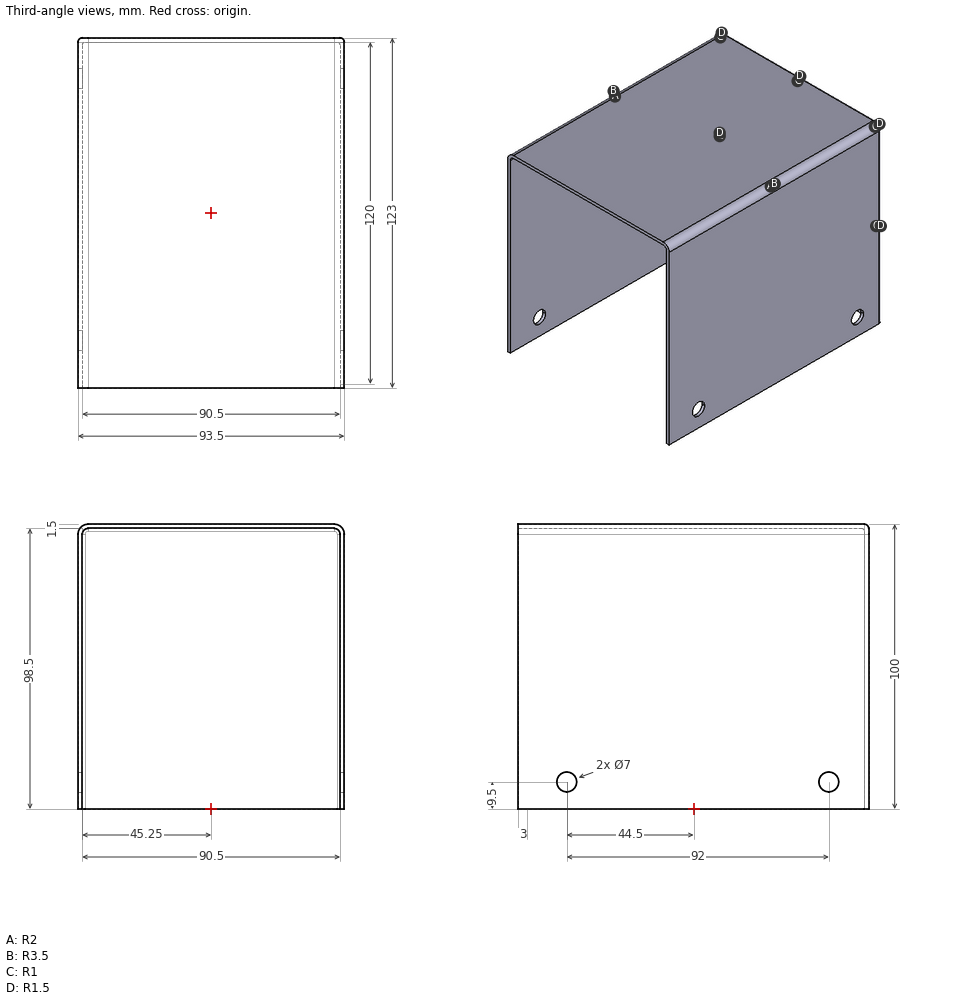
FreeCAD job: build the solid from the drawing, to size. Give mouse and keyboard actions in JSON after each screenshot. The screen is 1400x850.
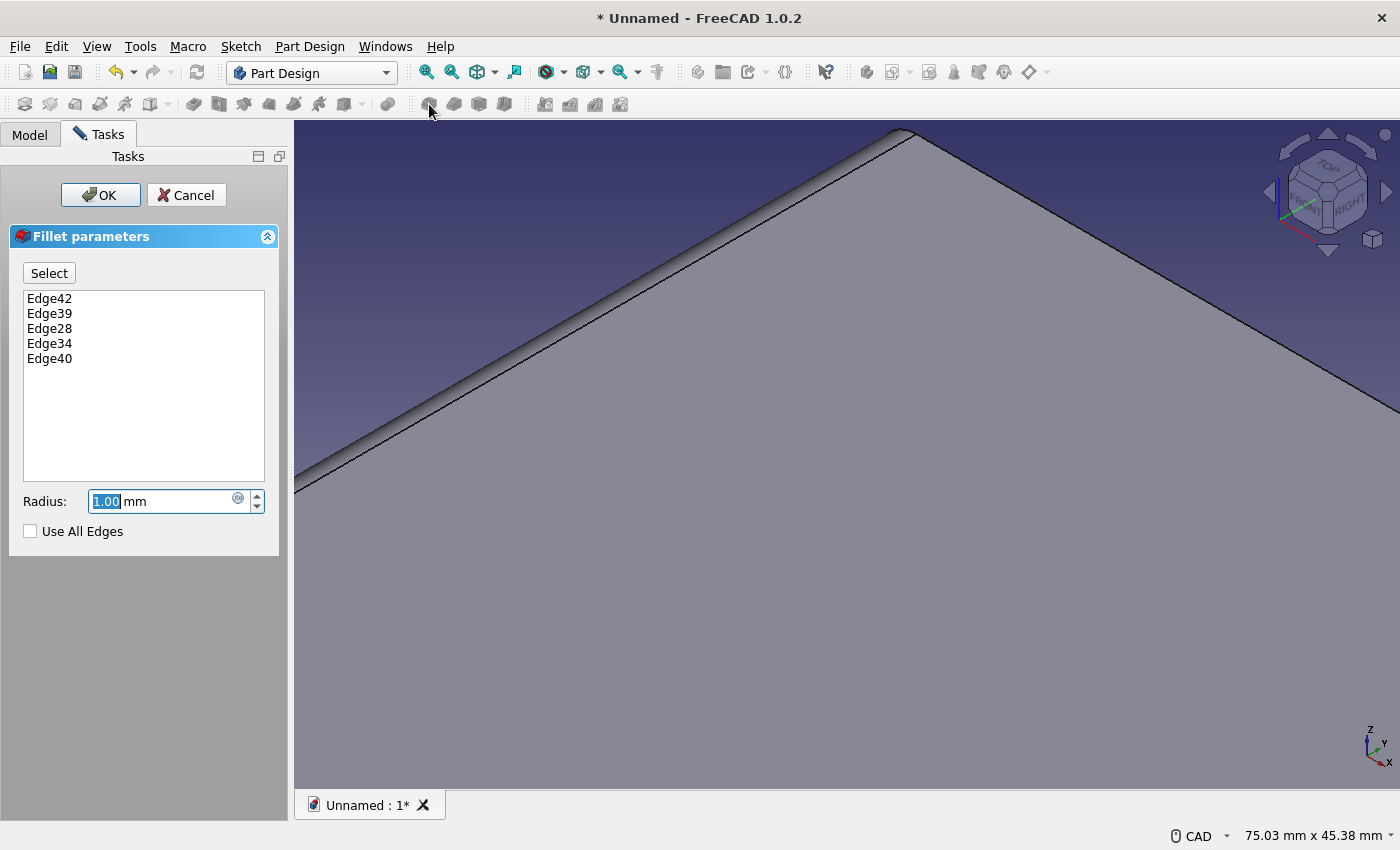
{"action": "type", "text": "1"}
{"action": "key", "text": "Tab"}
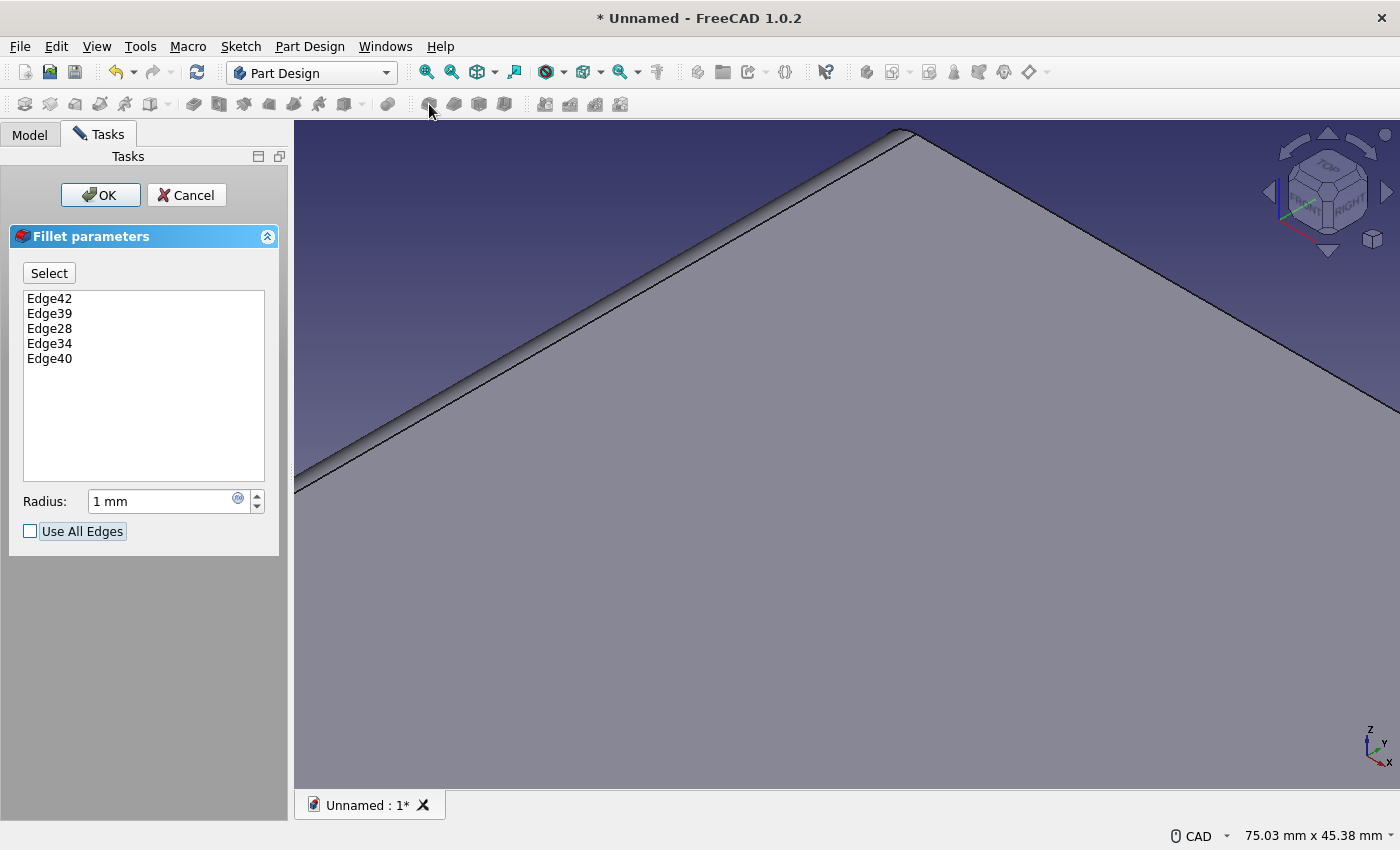
{"action": "left_click", "coordinate": [101, 195]}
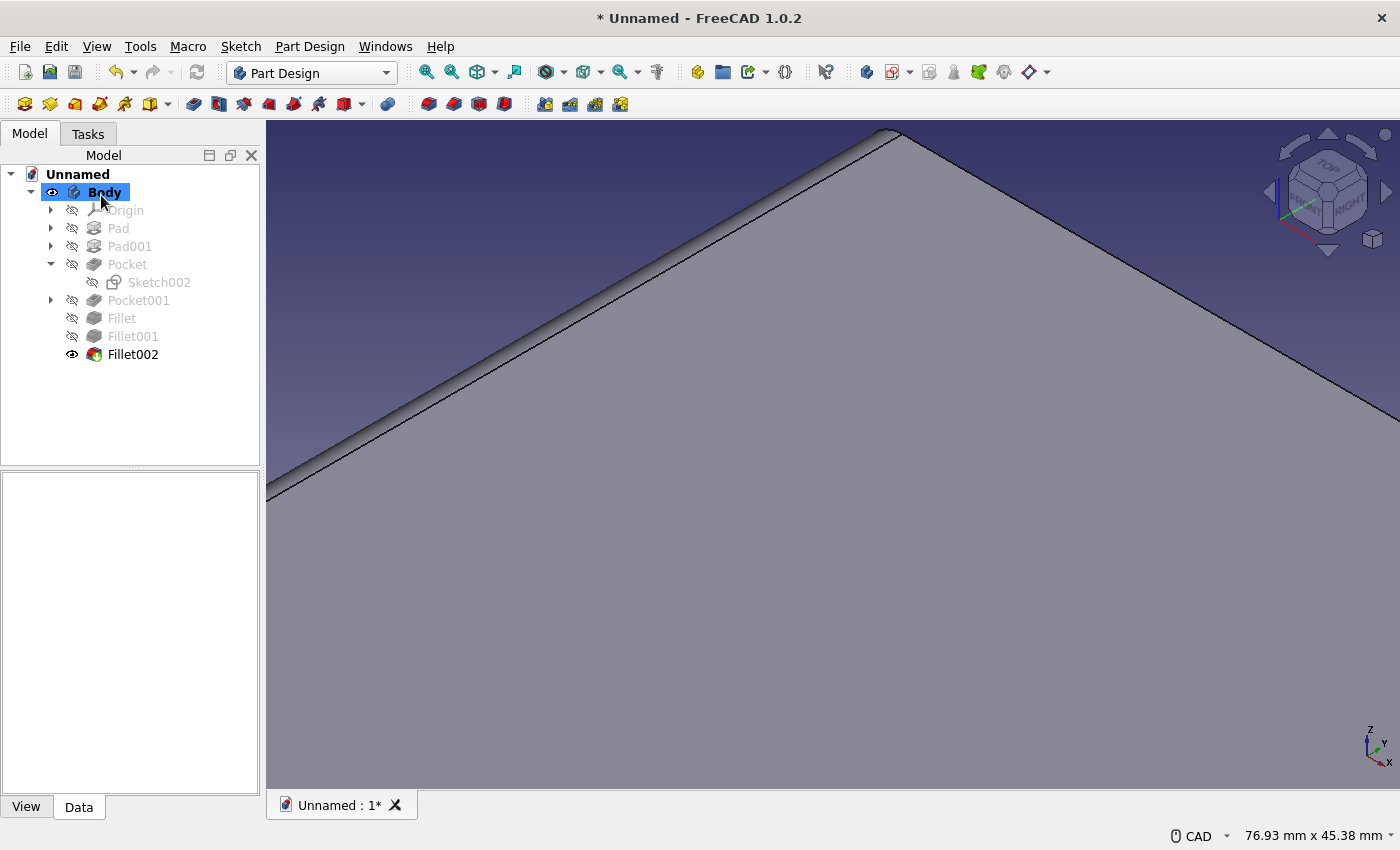
{"action": "left_click", "coordinate": [427, 72]}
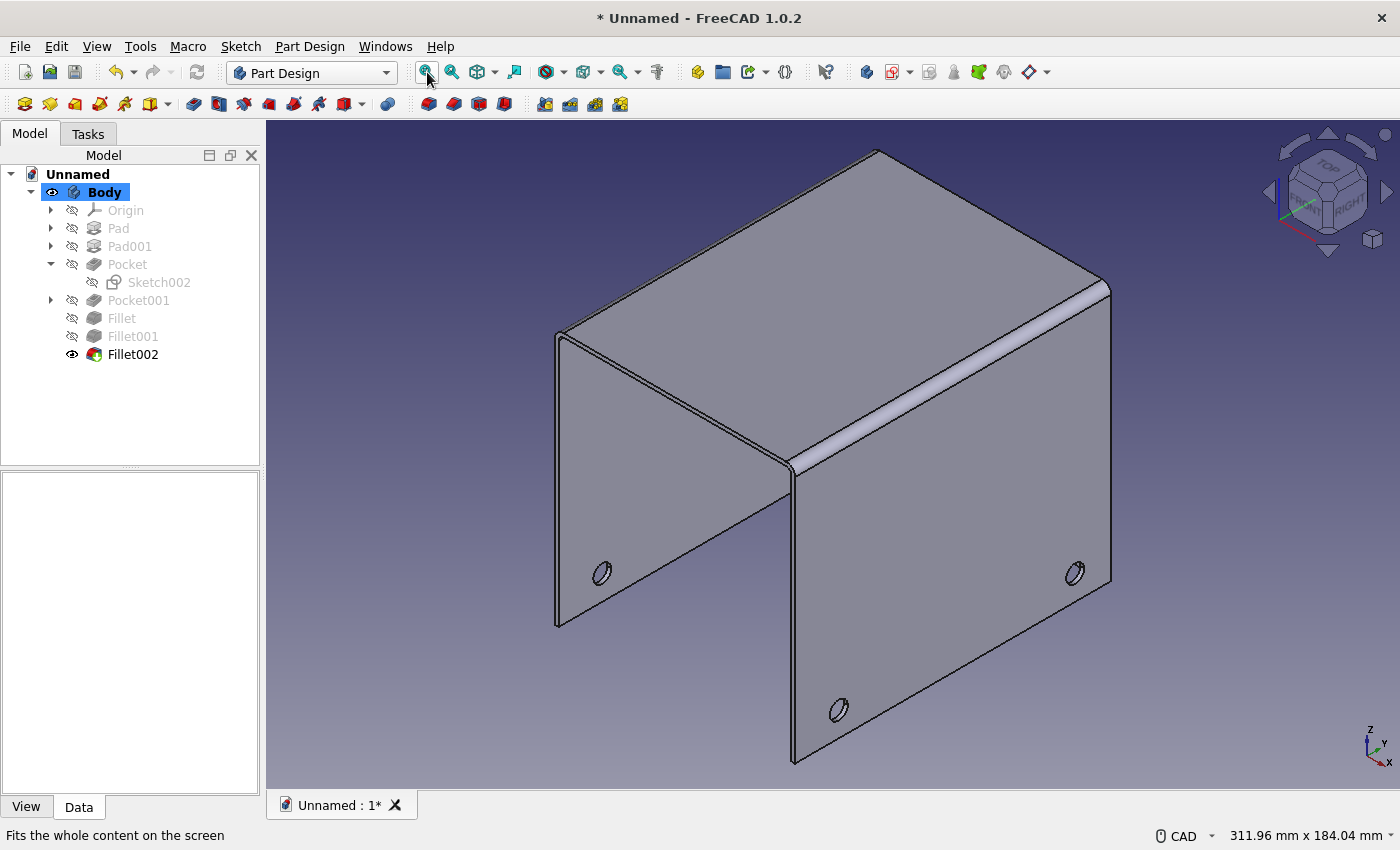
{"action": "left_click", "coordinate": [1111, 290]}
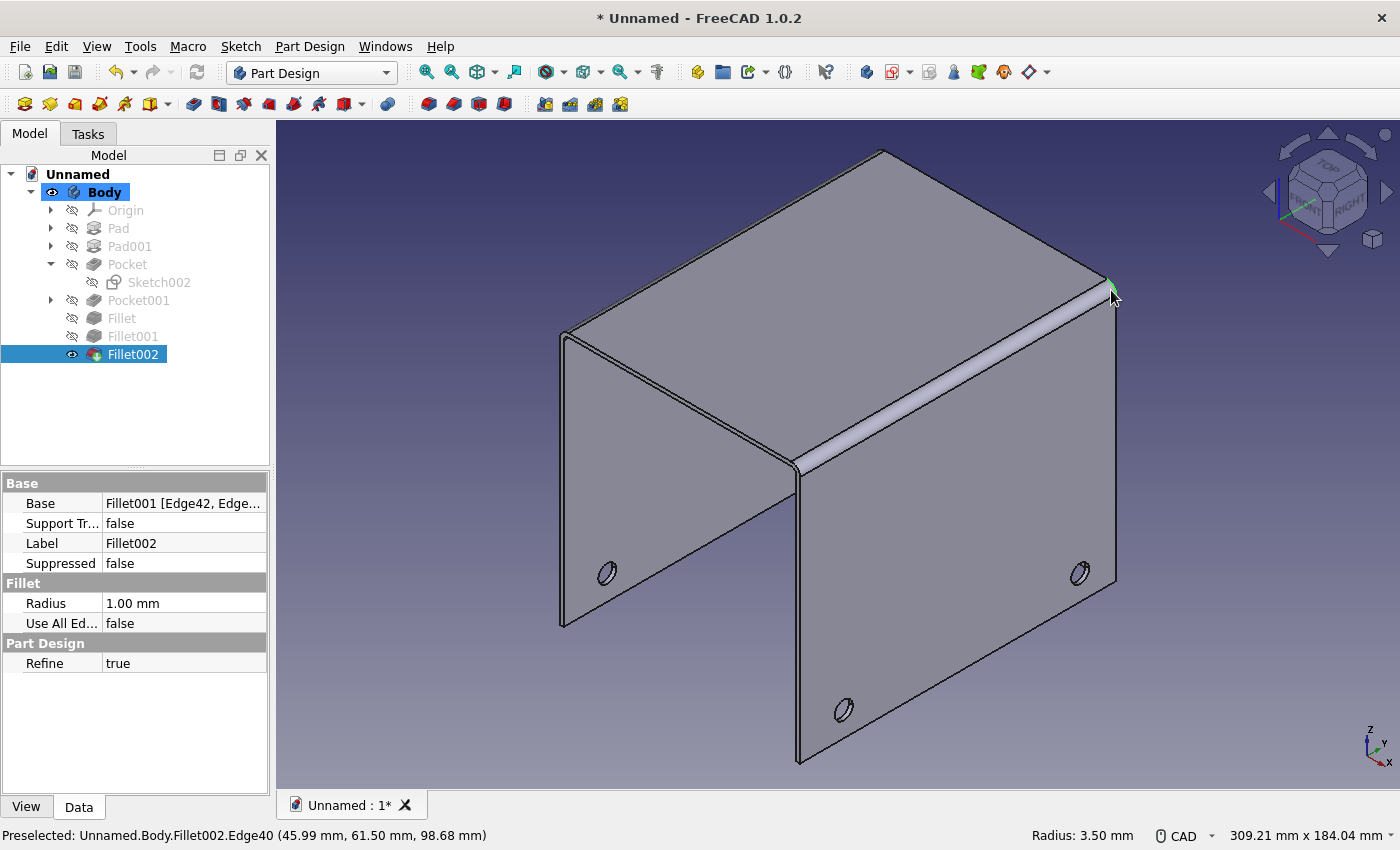
{"action": "key", "text": "2"}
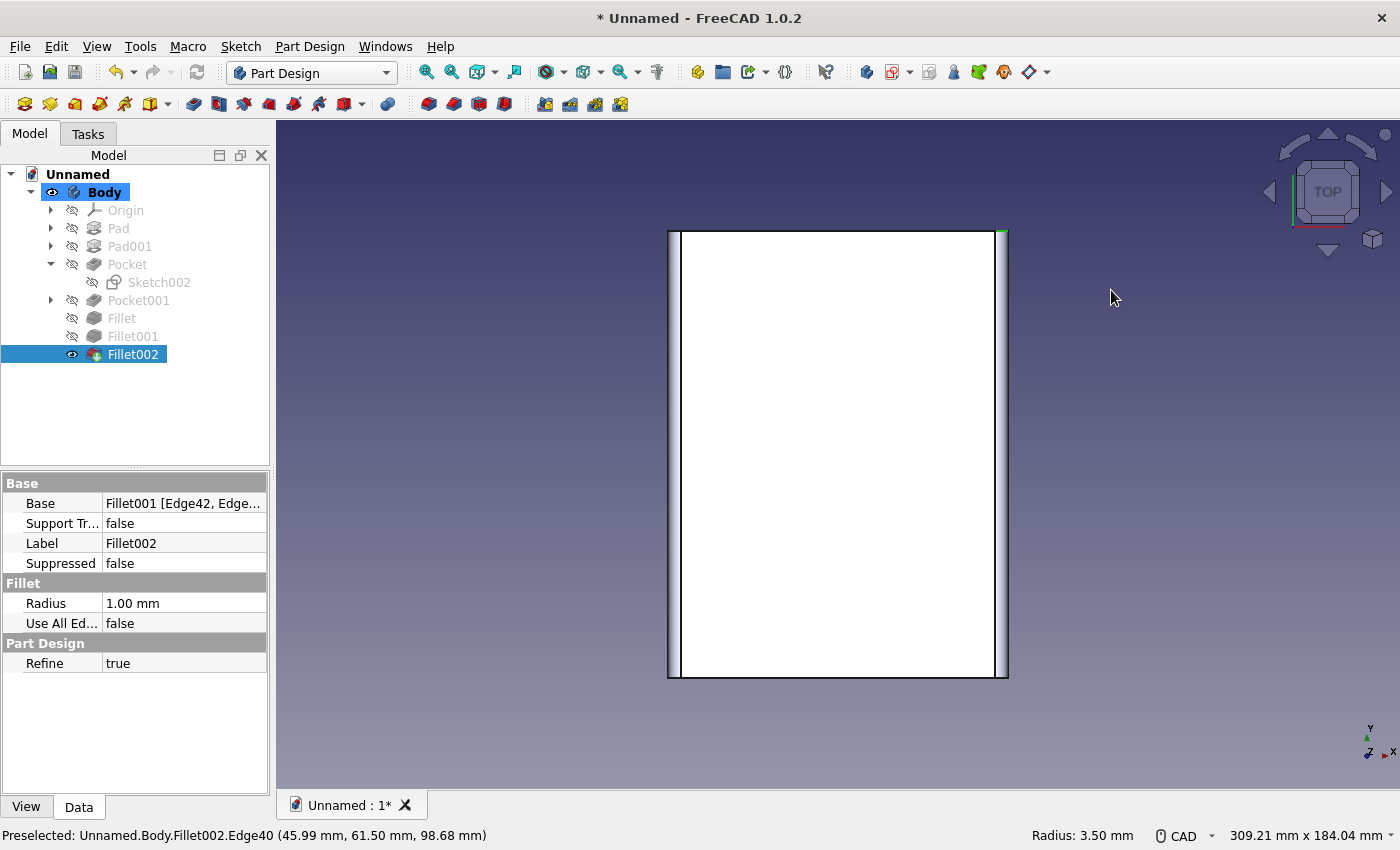
{"action": "left_click", "coordinate": [672, 230], "text": "ctrl"}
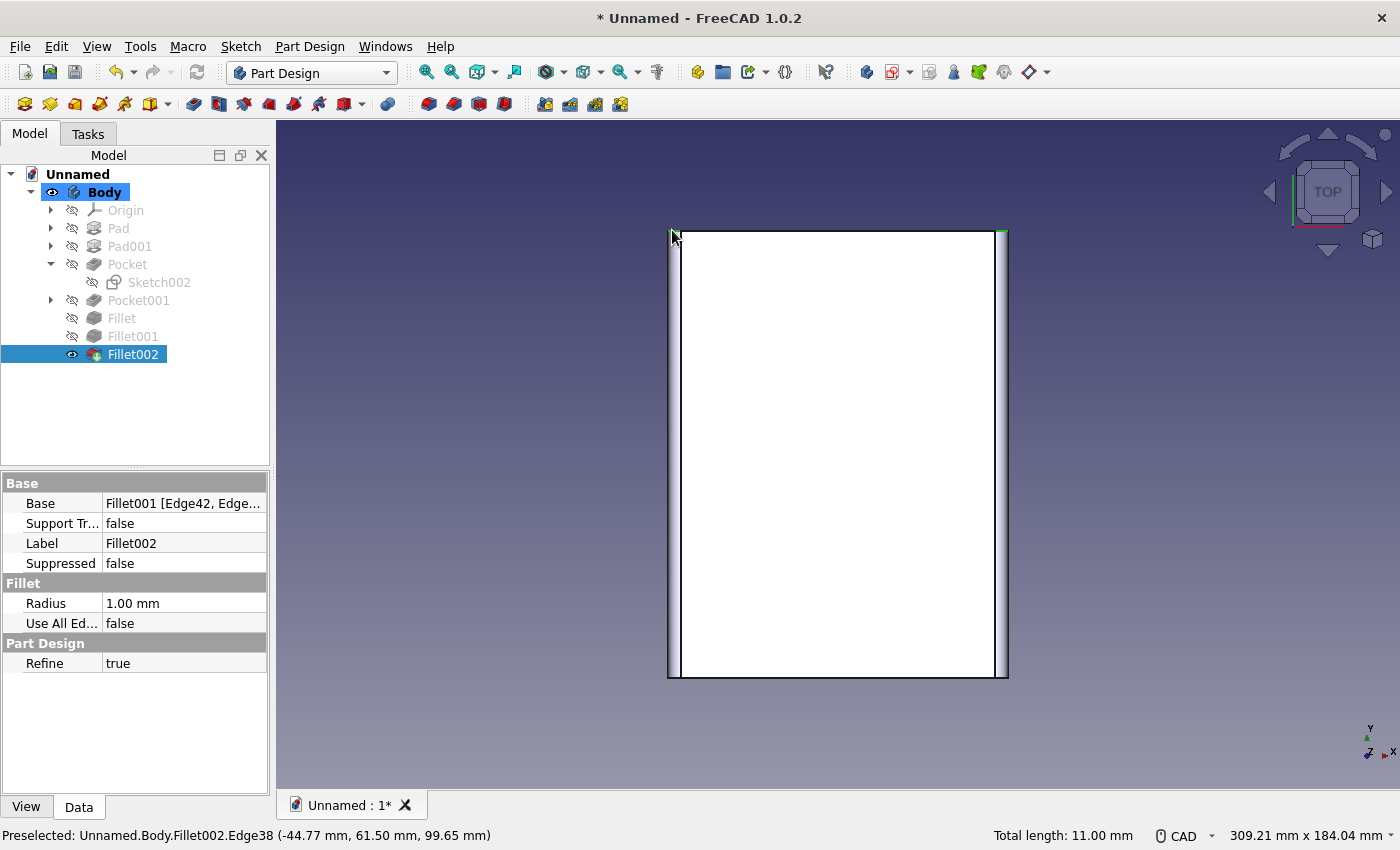
{"action": "left_click", "coordinate": [838, 230], "text": "ctrl"}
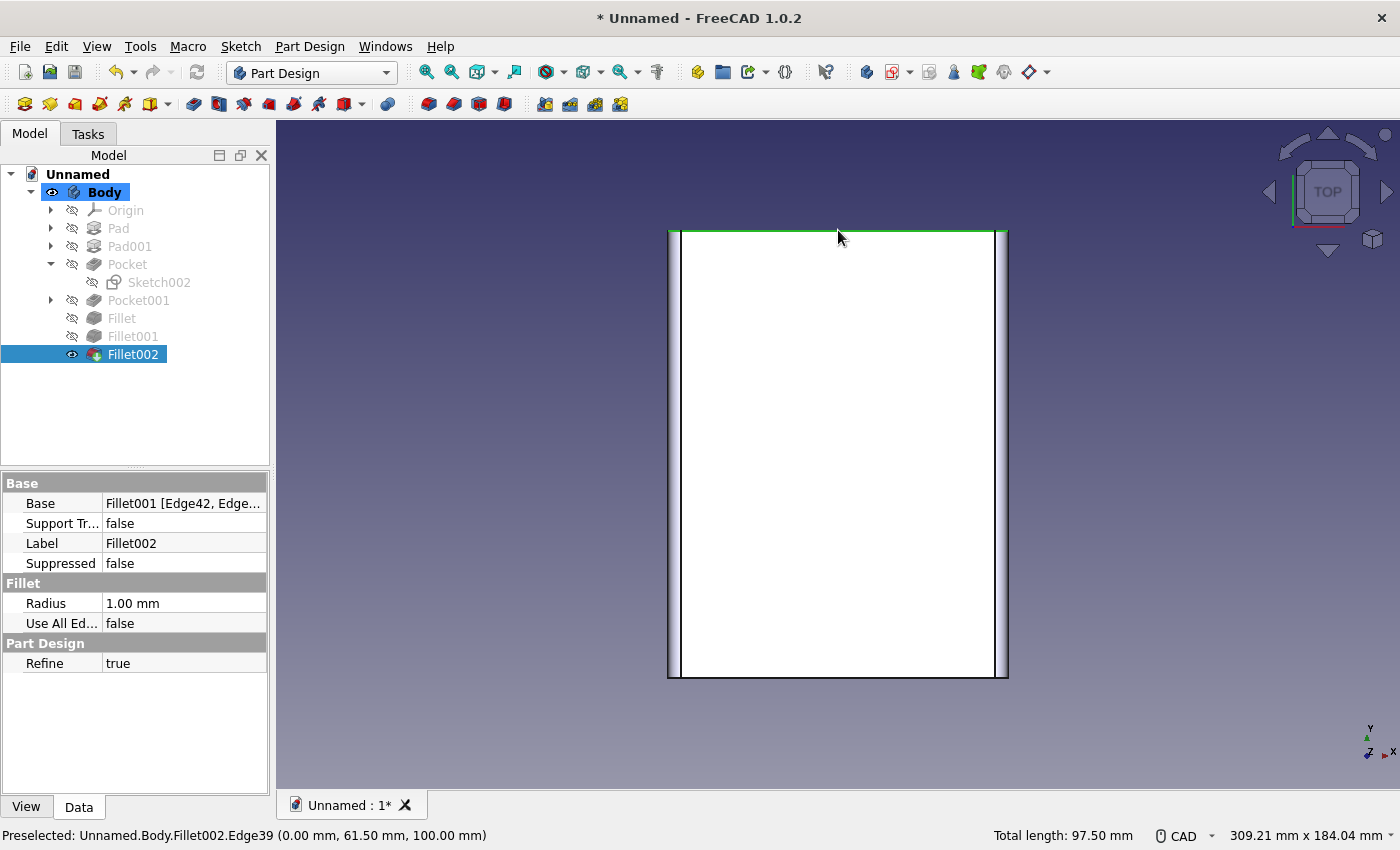
{"action": "key", "text": "0"}